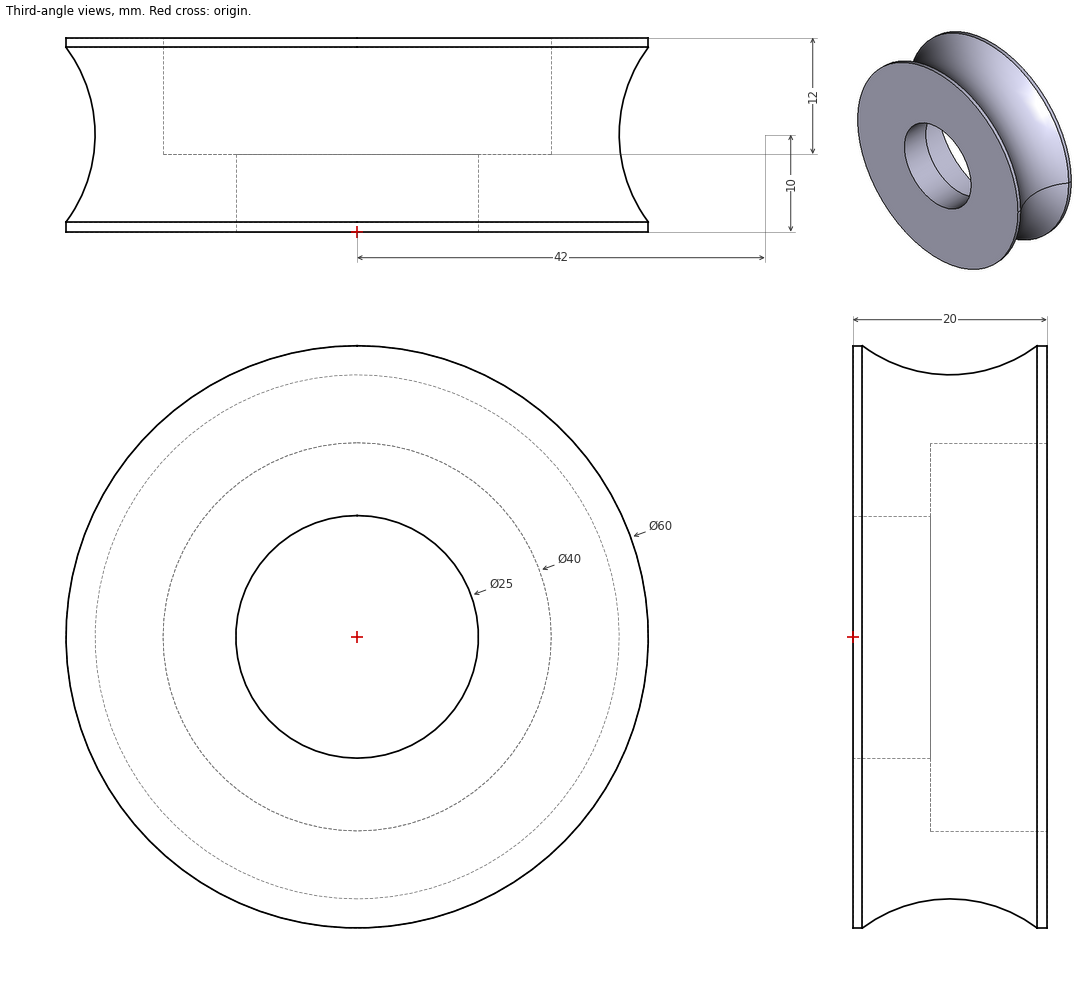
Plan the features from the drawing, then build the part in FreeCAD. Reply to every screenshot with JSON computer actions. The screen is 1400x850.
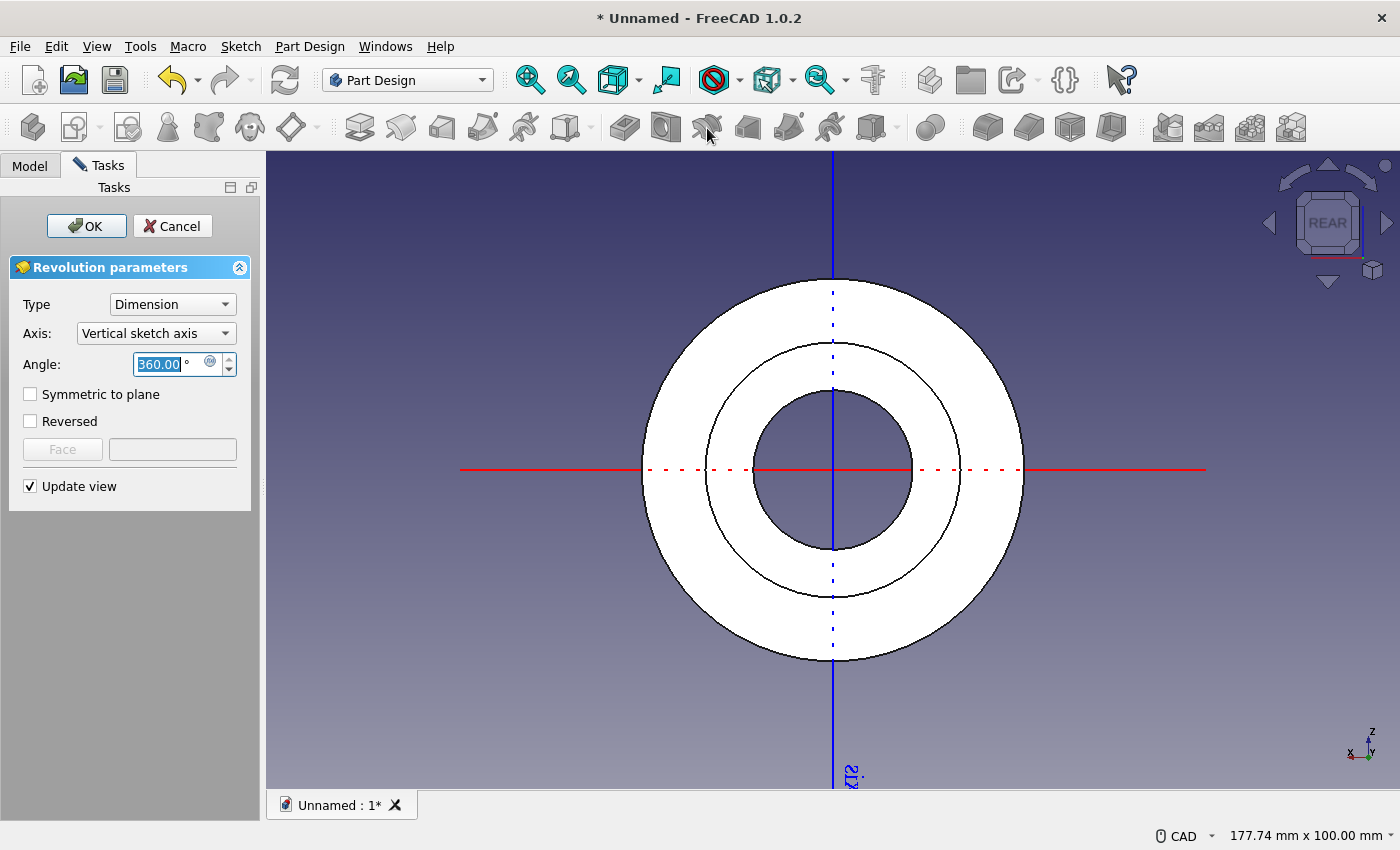
{"action": "left_click", "coordinate": [87, 226]}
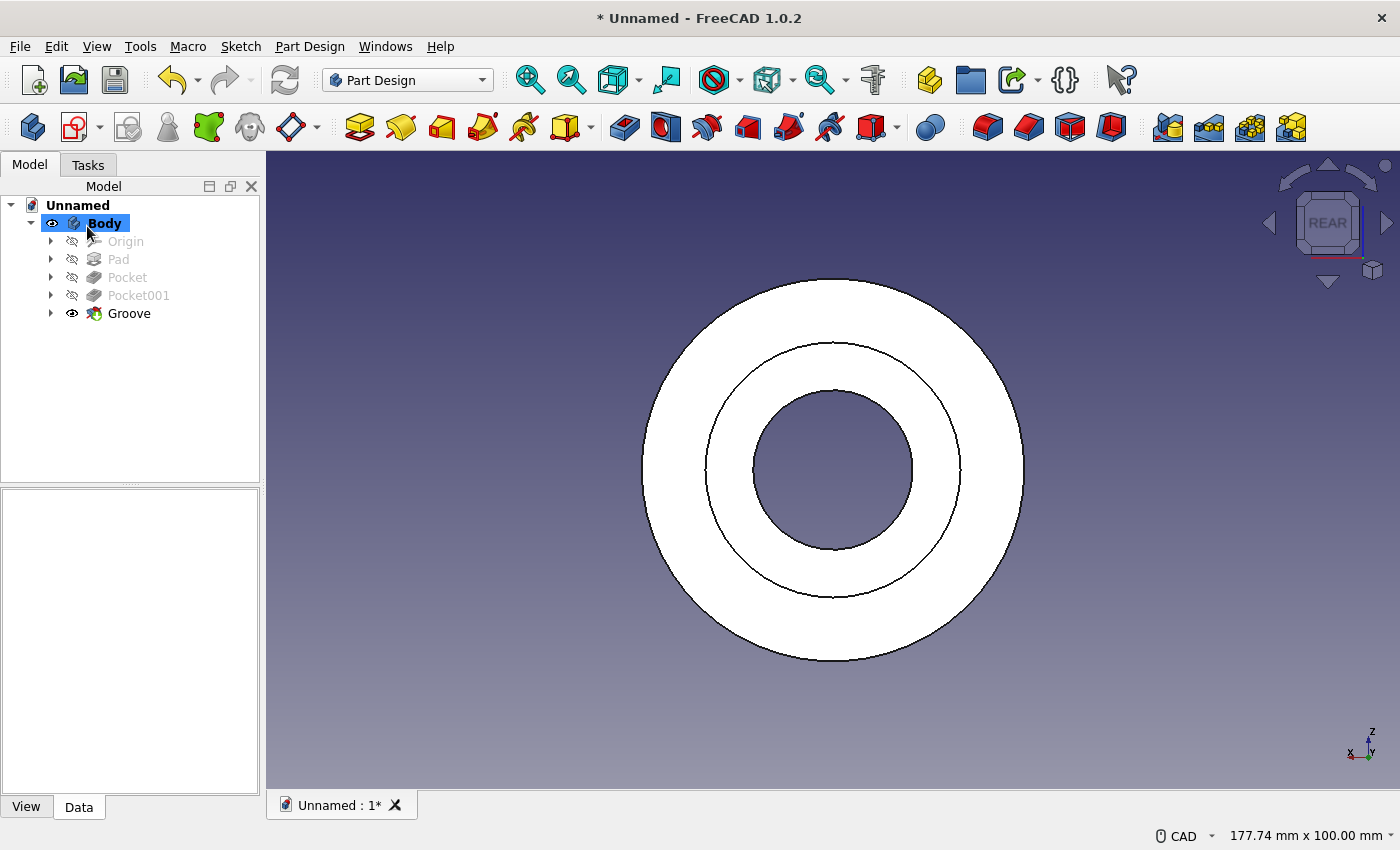
{"action": "key", "text": "0"}